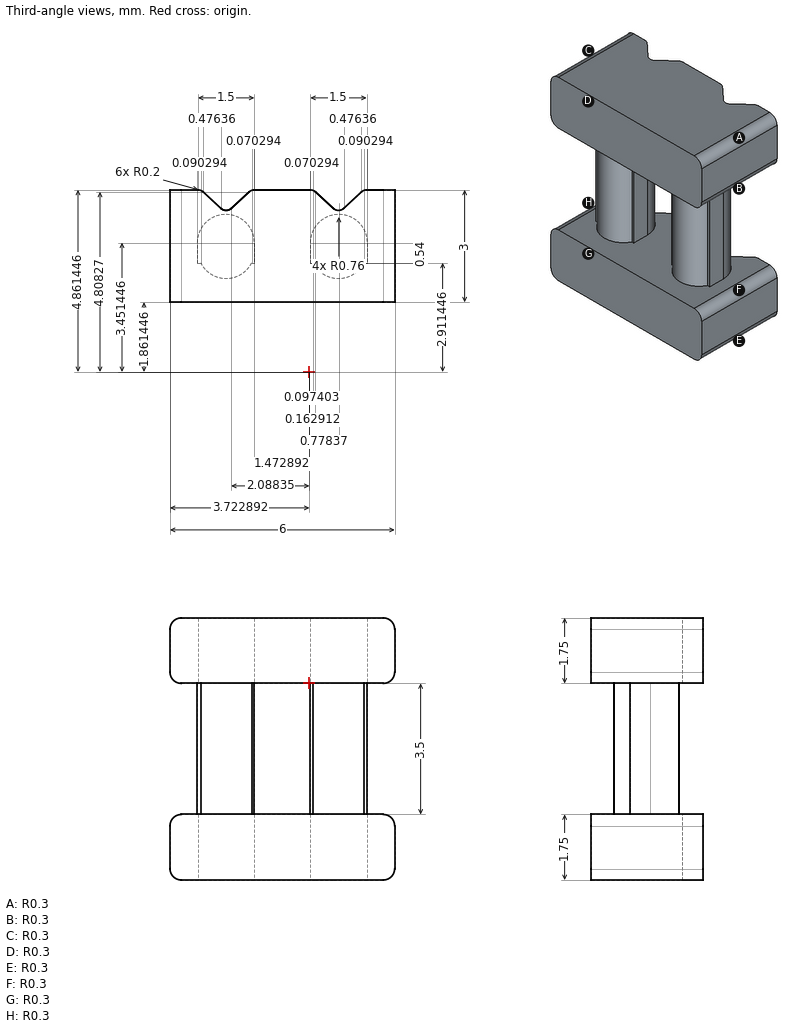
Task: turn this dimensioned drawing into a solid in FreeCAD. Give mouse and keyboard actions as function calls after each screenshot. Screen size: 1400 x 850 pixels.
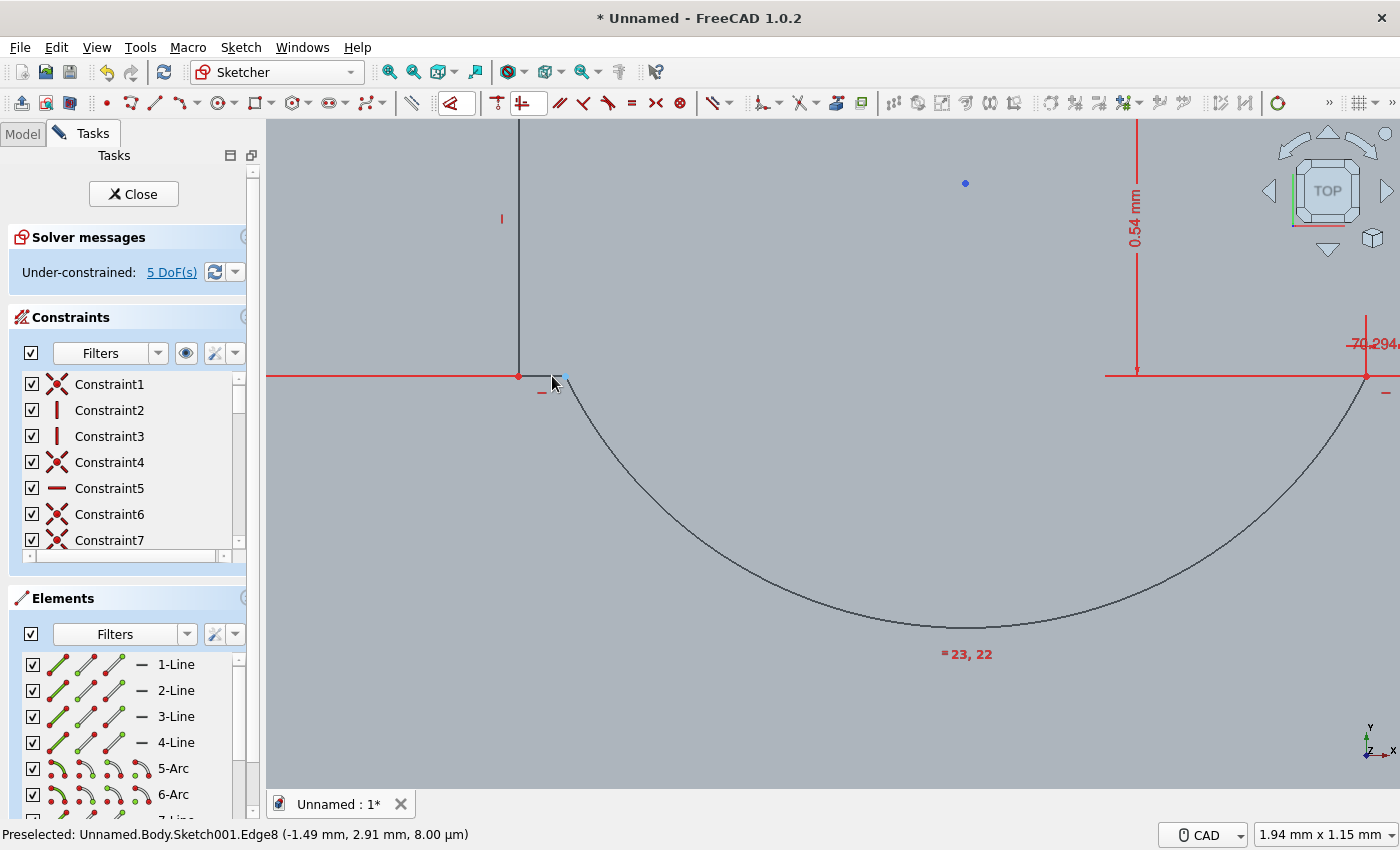
click(552, 376)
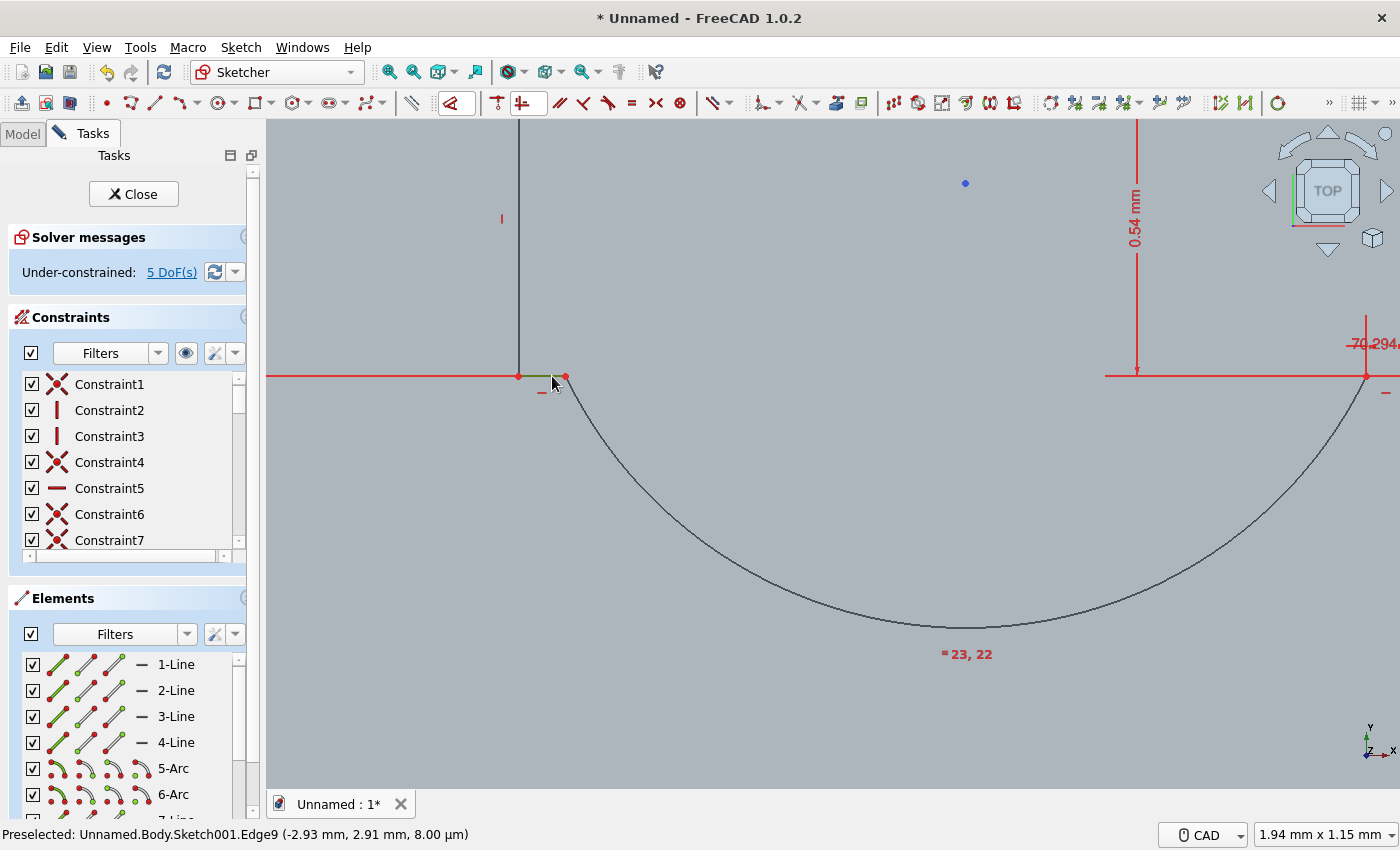
click(470, 104)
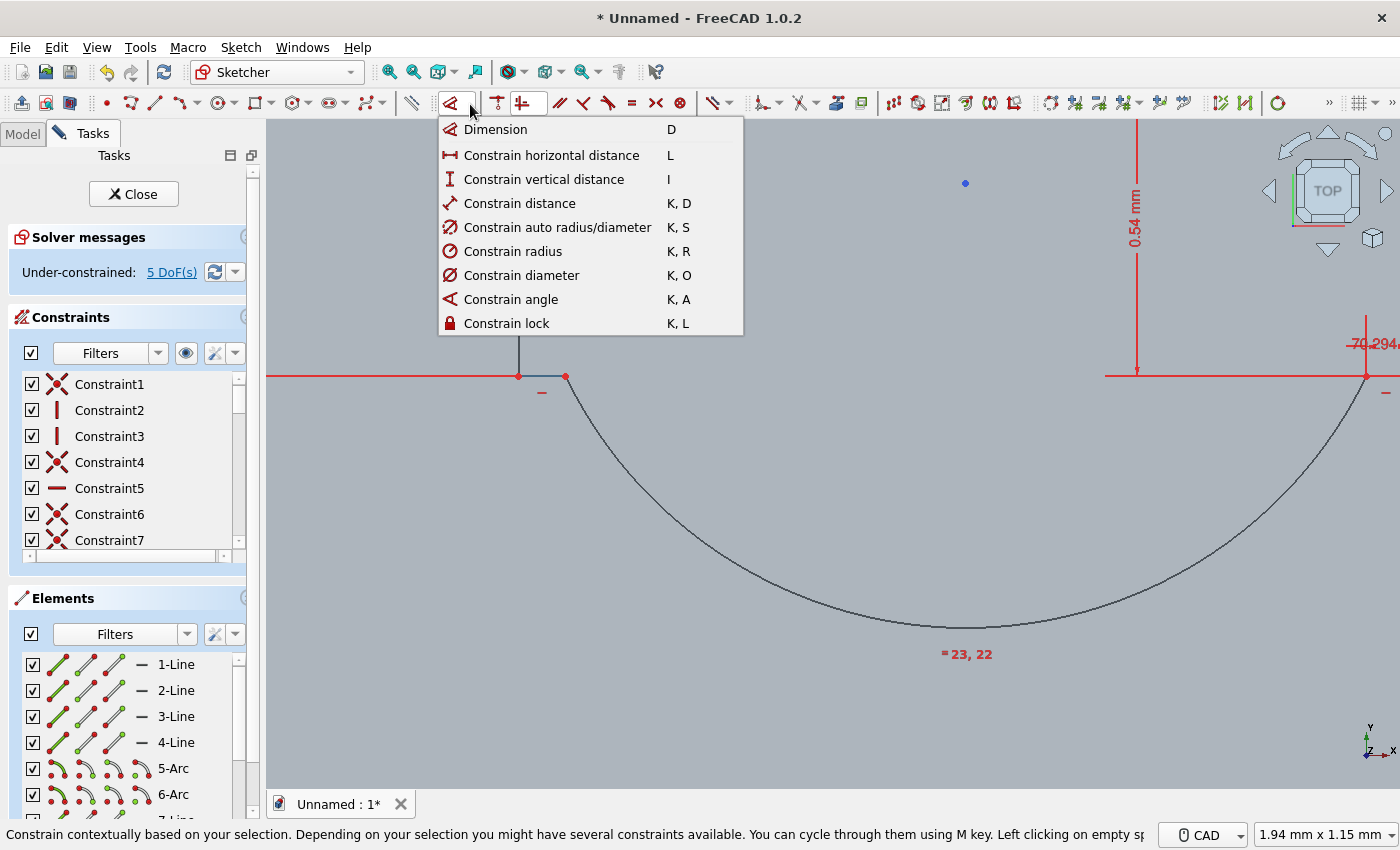
click(591, 155)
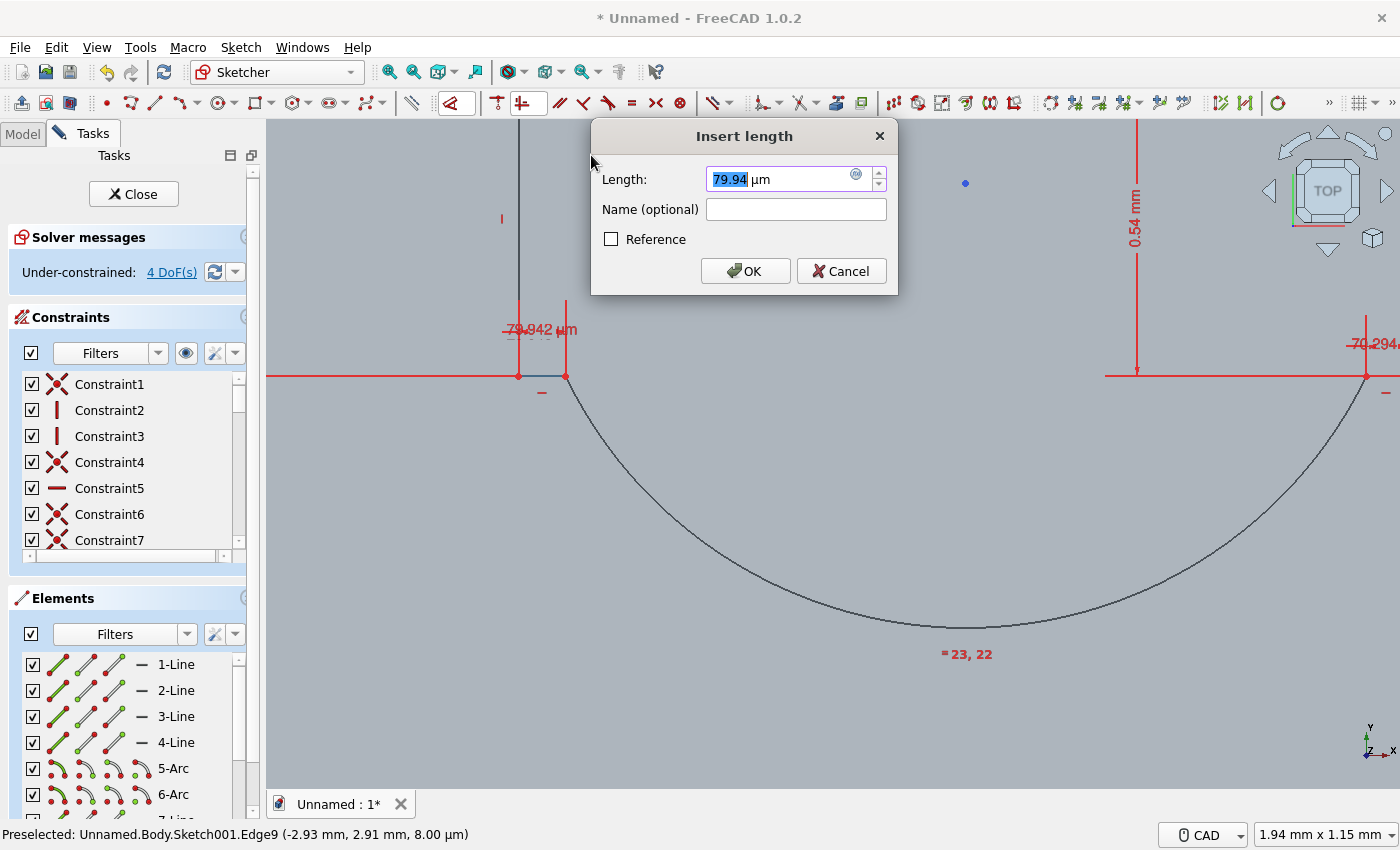
key(ctrl+a)
text(0.090294 mm)
key(Return)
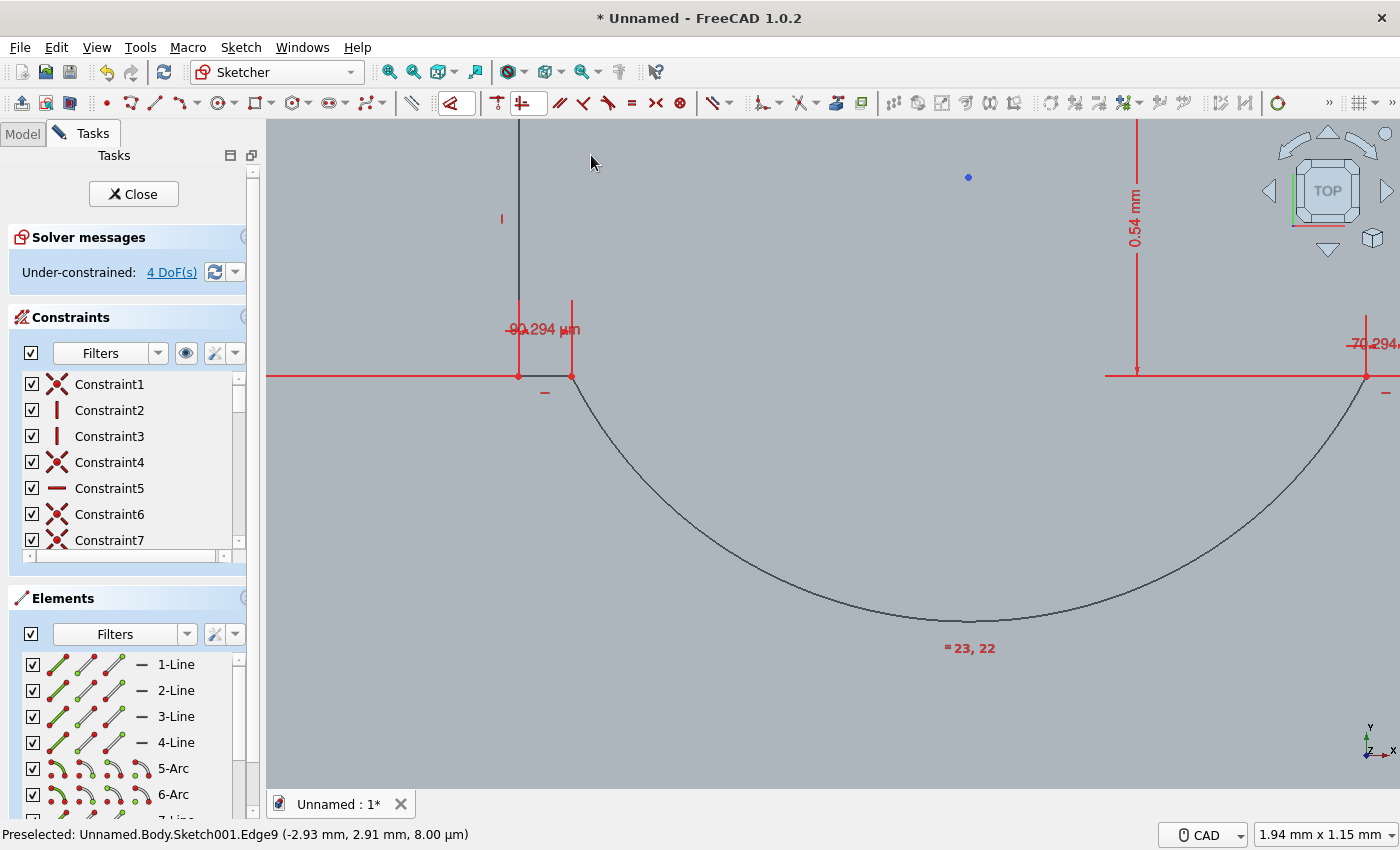
scroll(551, 376, down, 9)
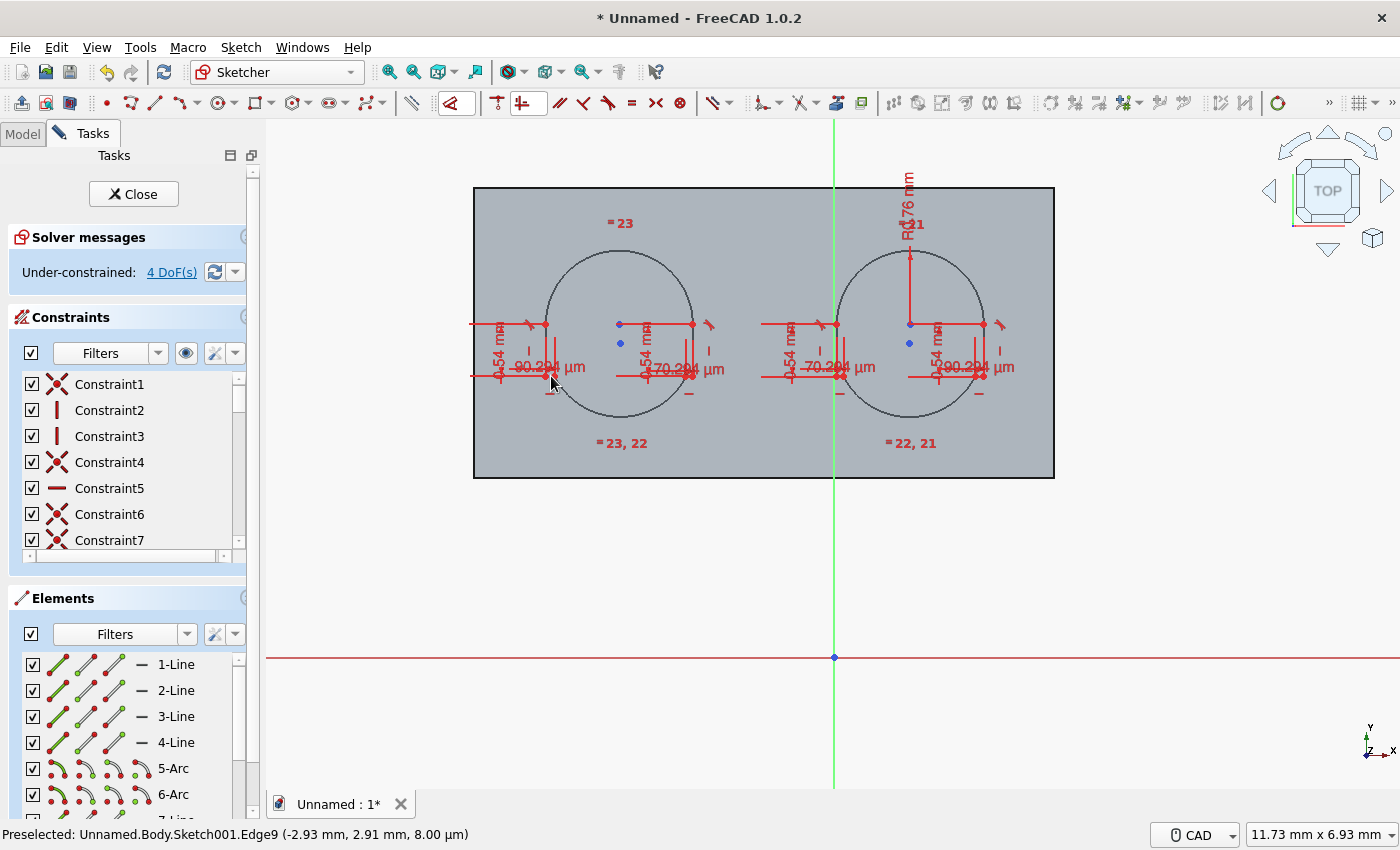
scroll(844, 377, up, 8)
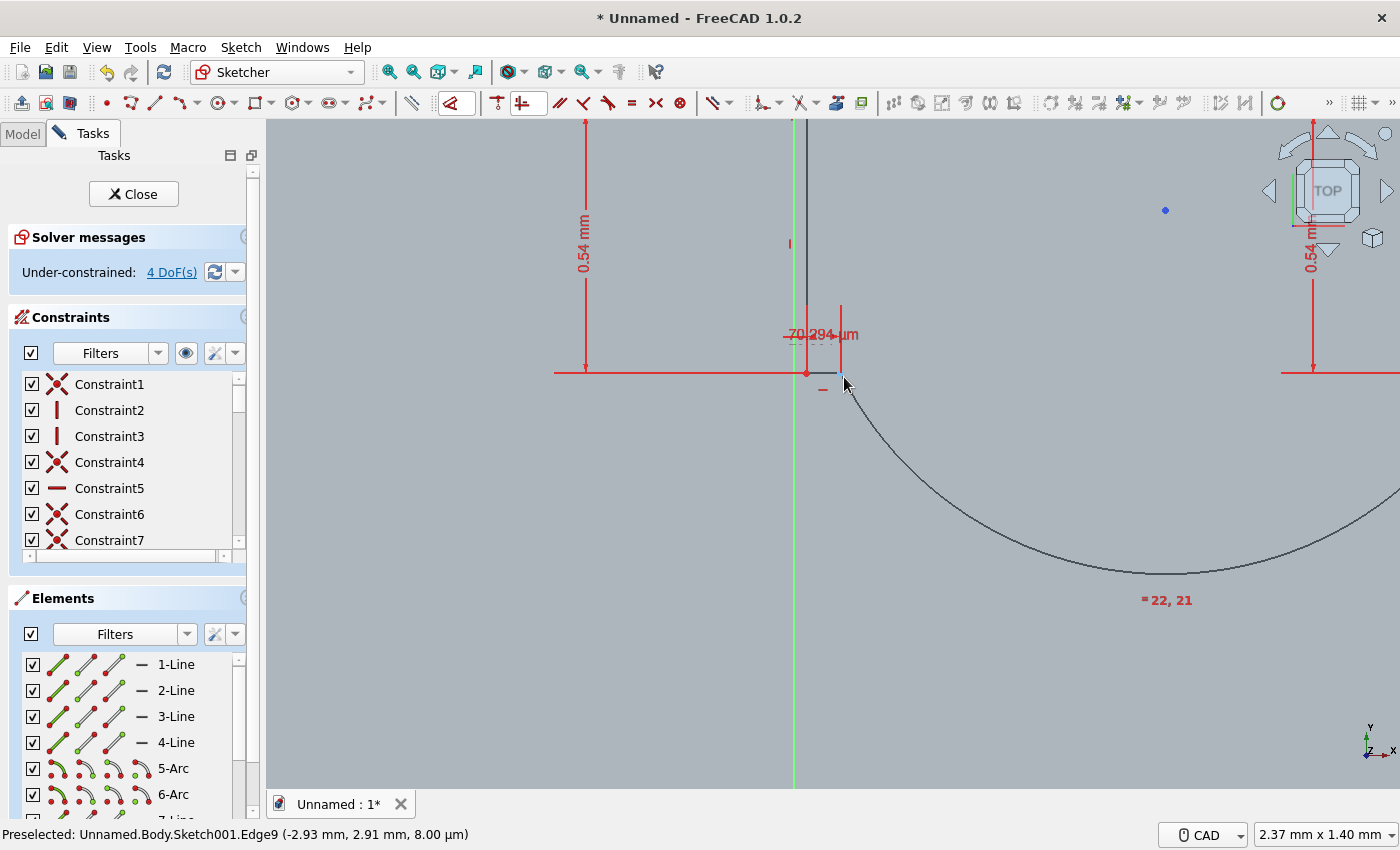
click(841, 373)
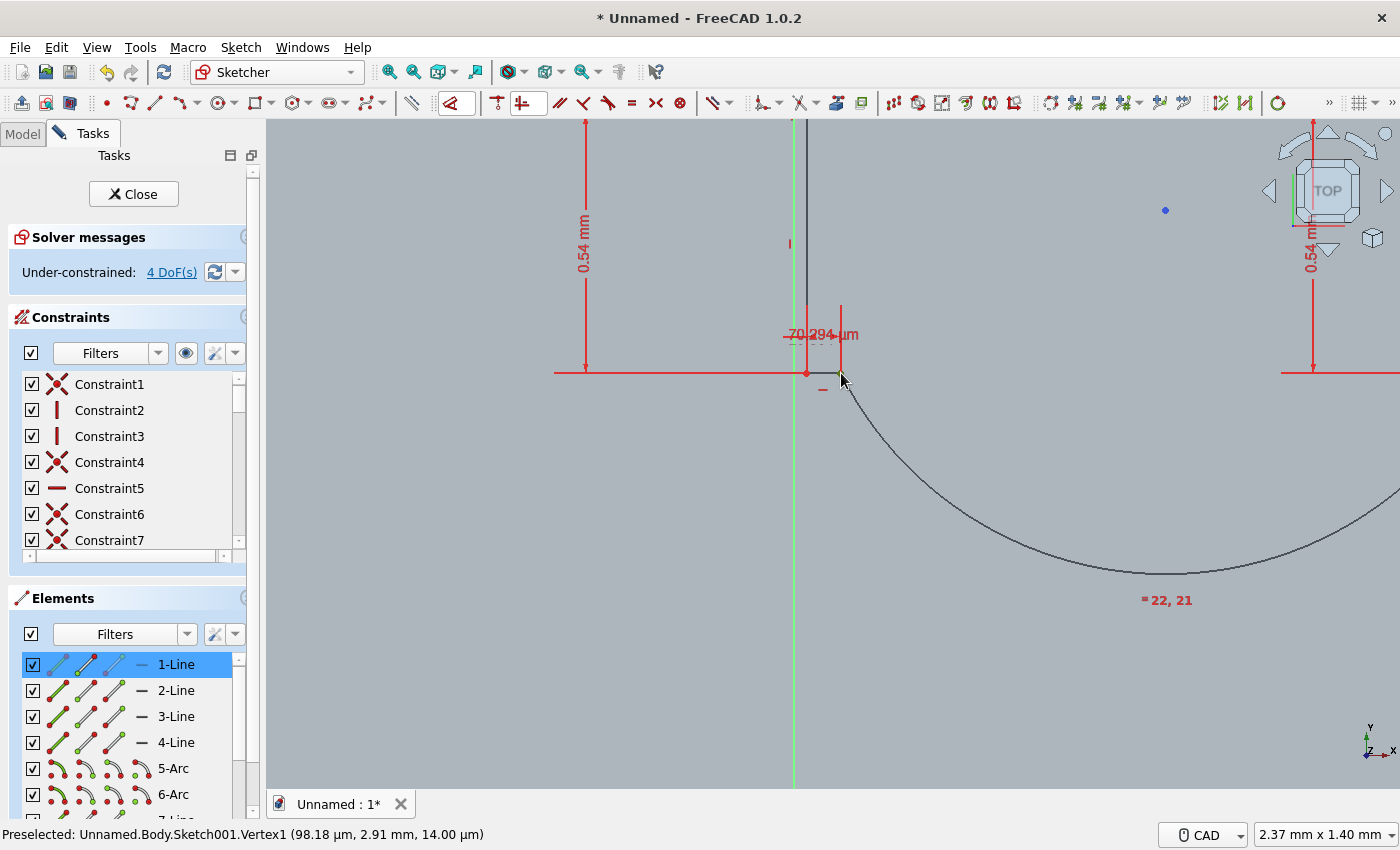
click(470, 104)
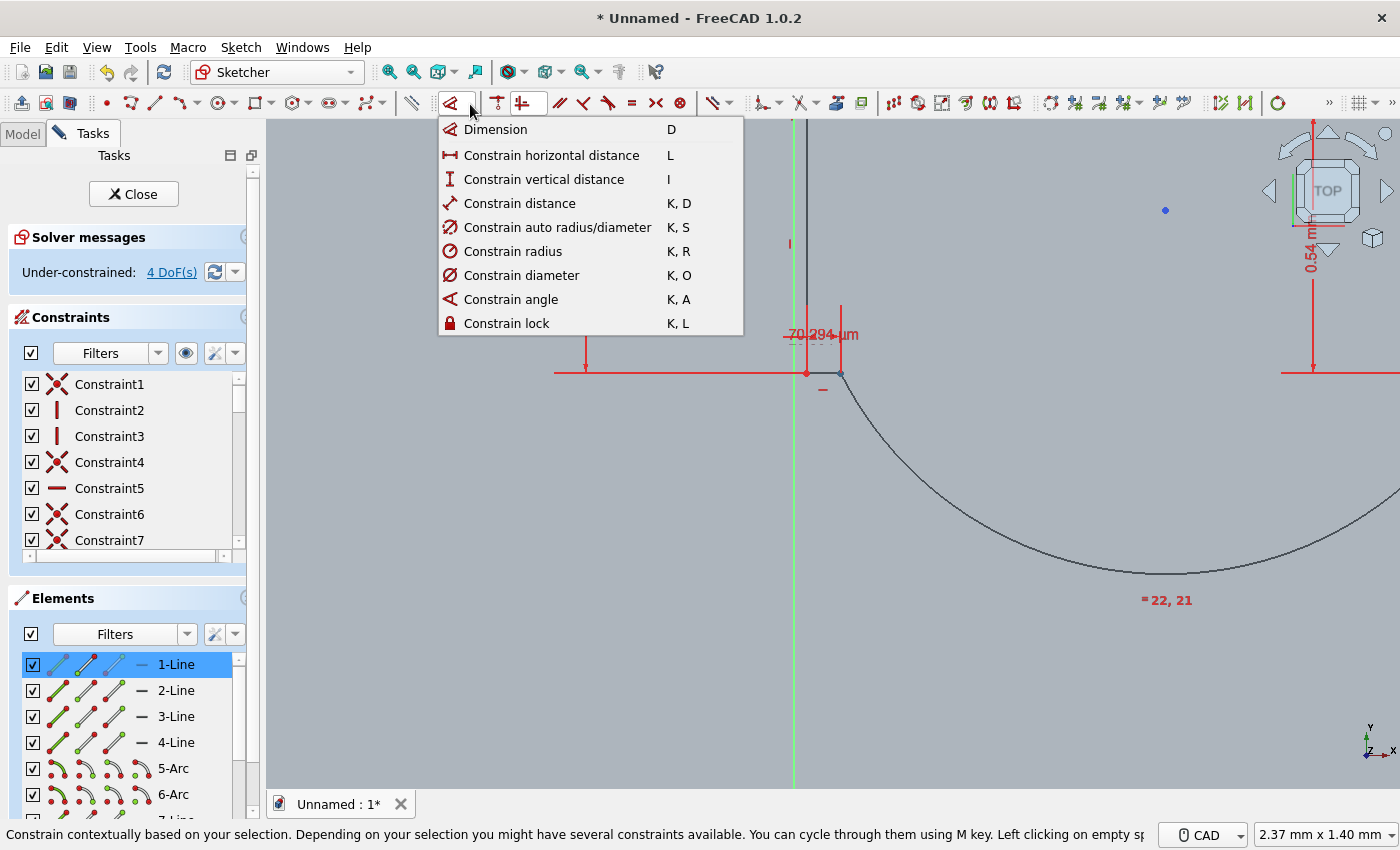
click(591, 155)